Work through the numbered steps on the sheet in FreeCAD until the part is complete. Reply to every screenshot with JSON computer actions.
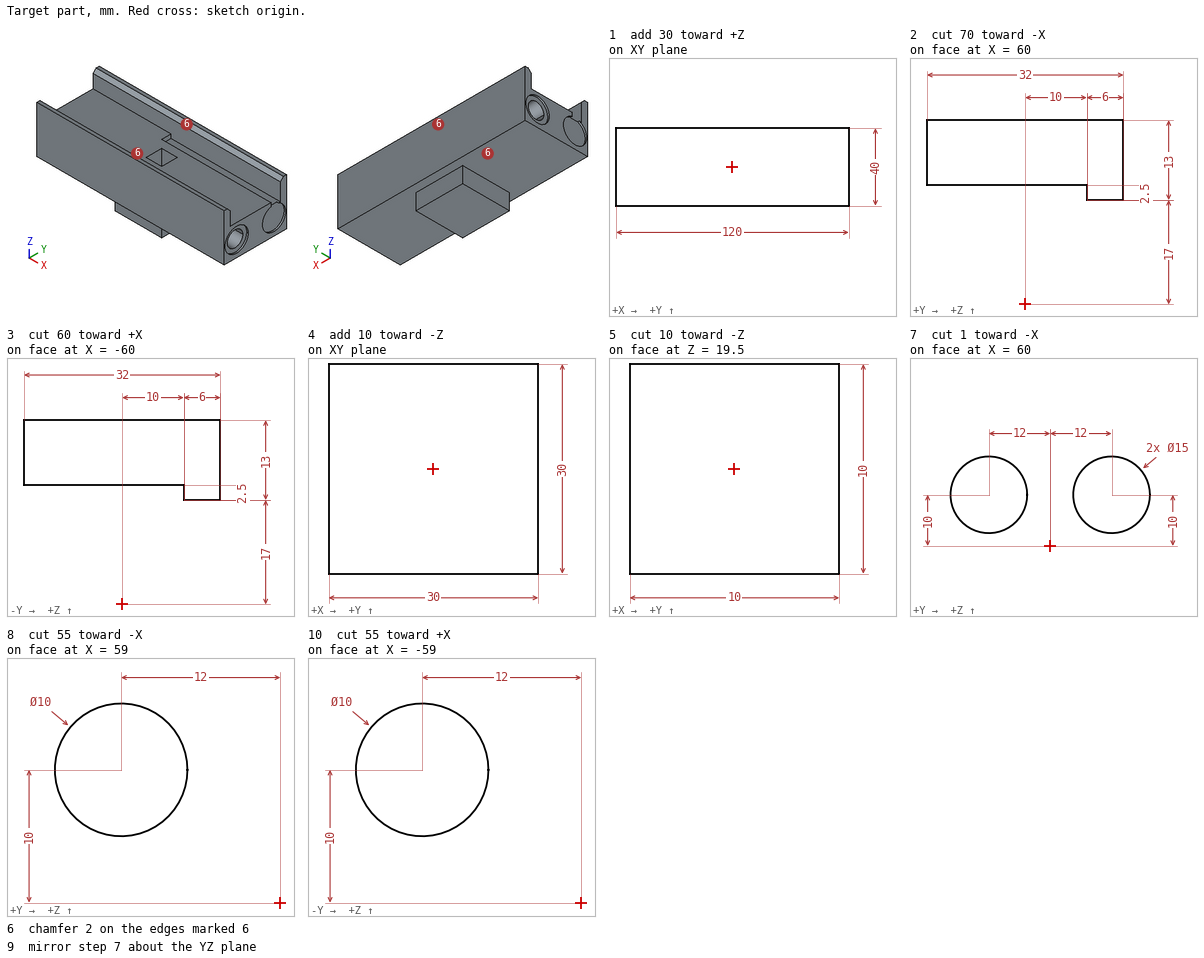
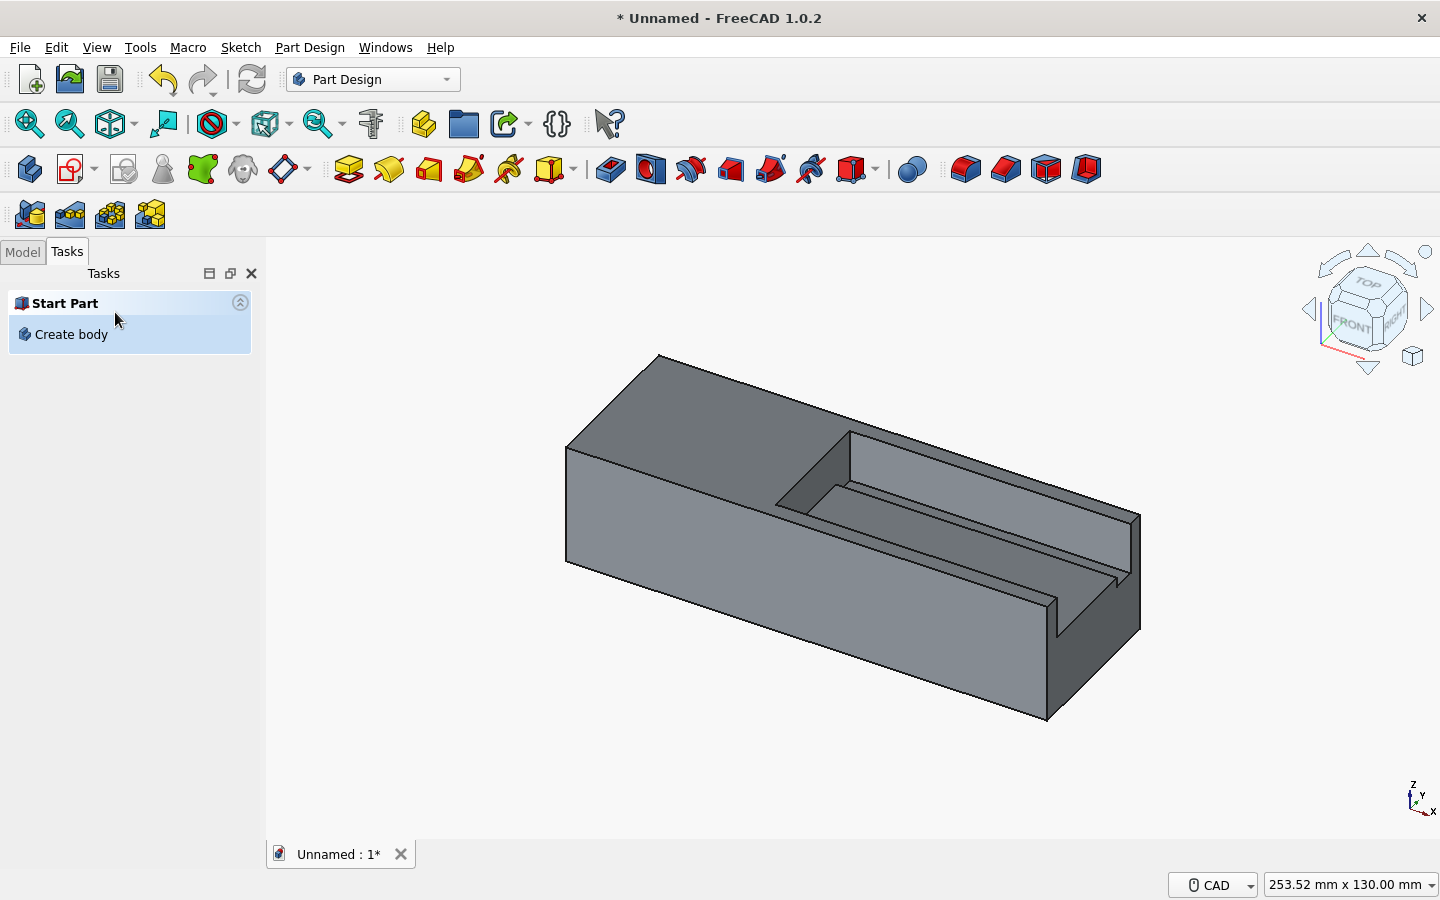
{"action": "key", "text": "6"}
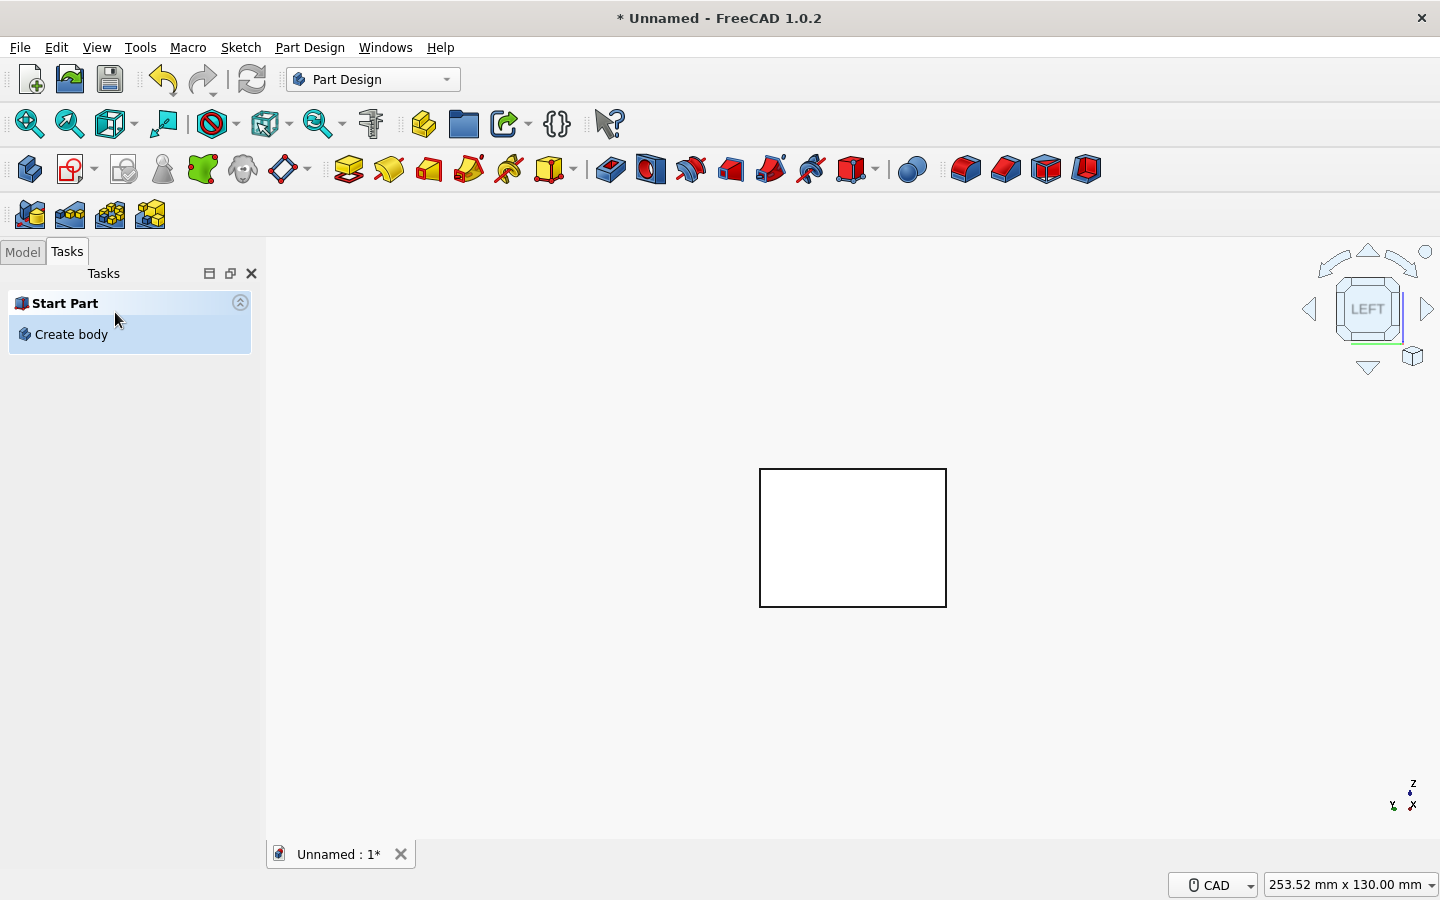
{"action": "left_click", "coordinate": [30, 124]}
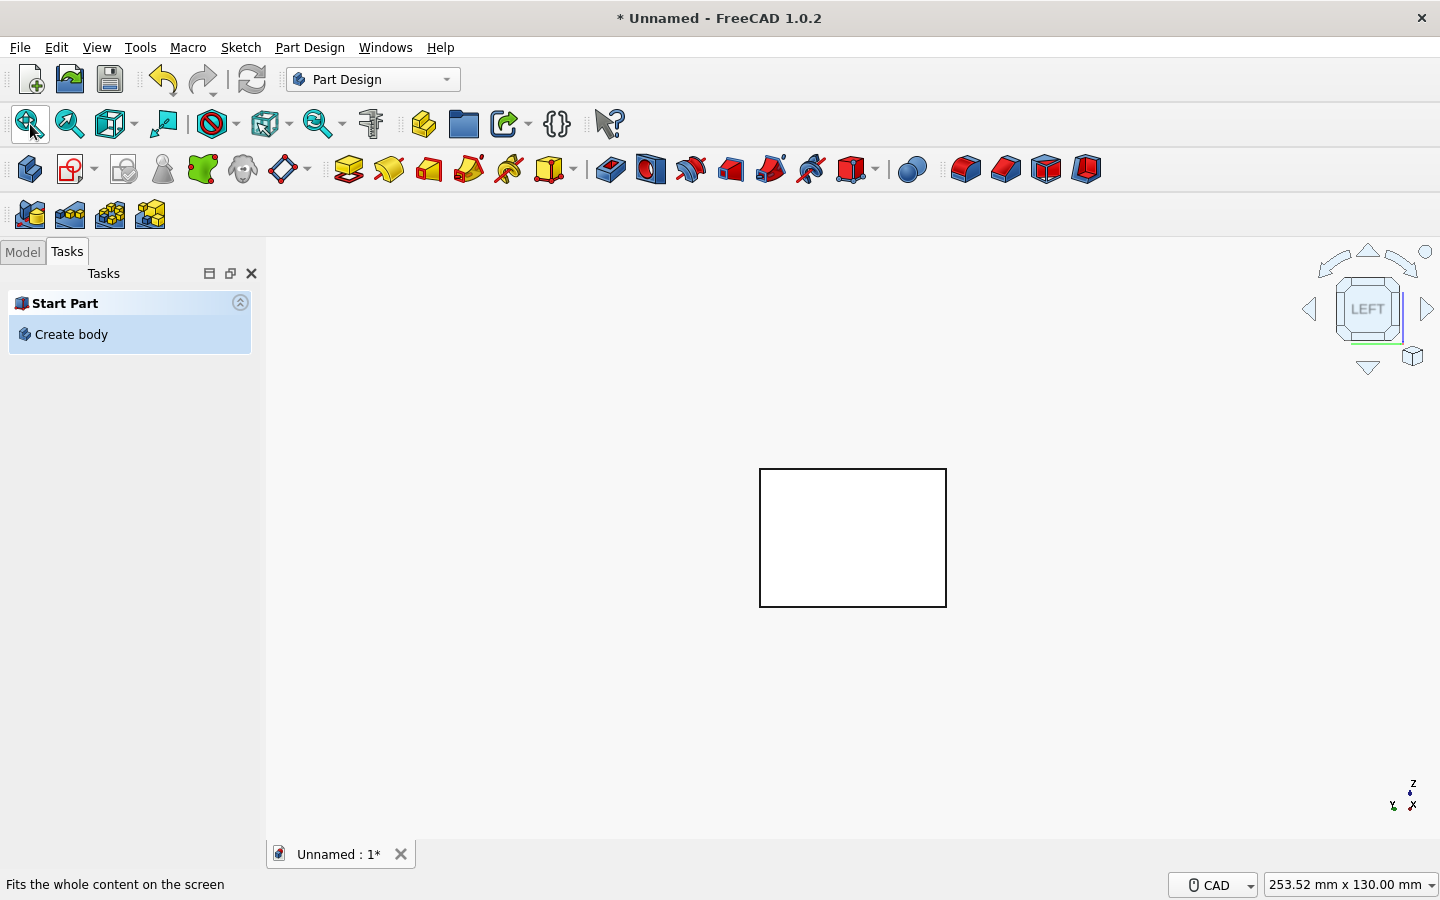
{"action": "left_click", "coordinate": [853, 537]}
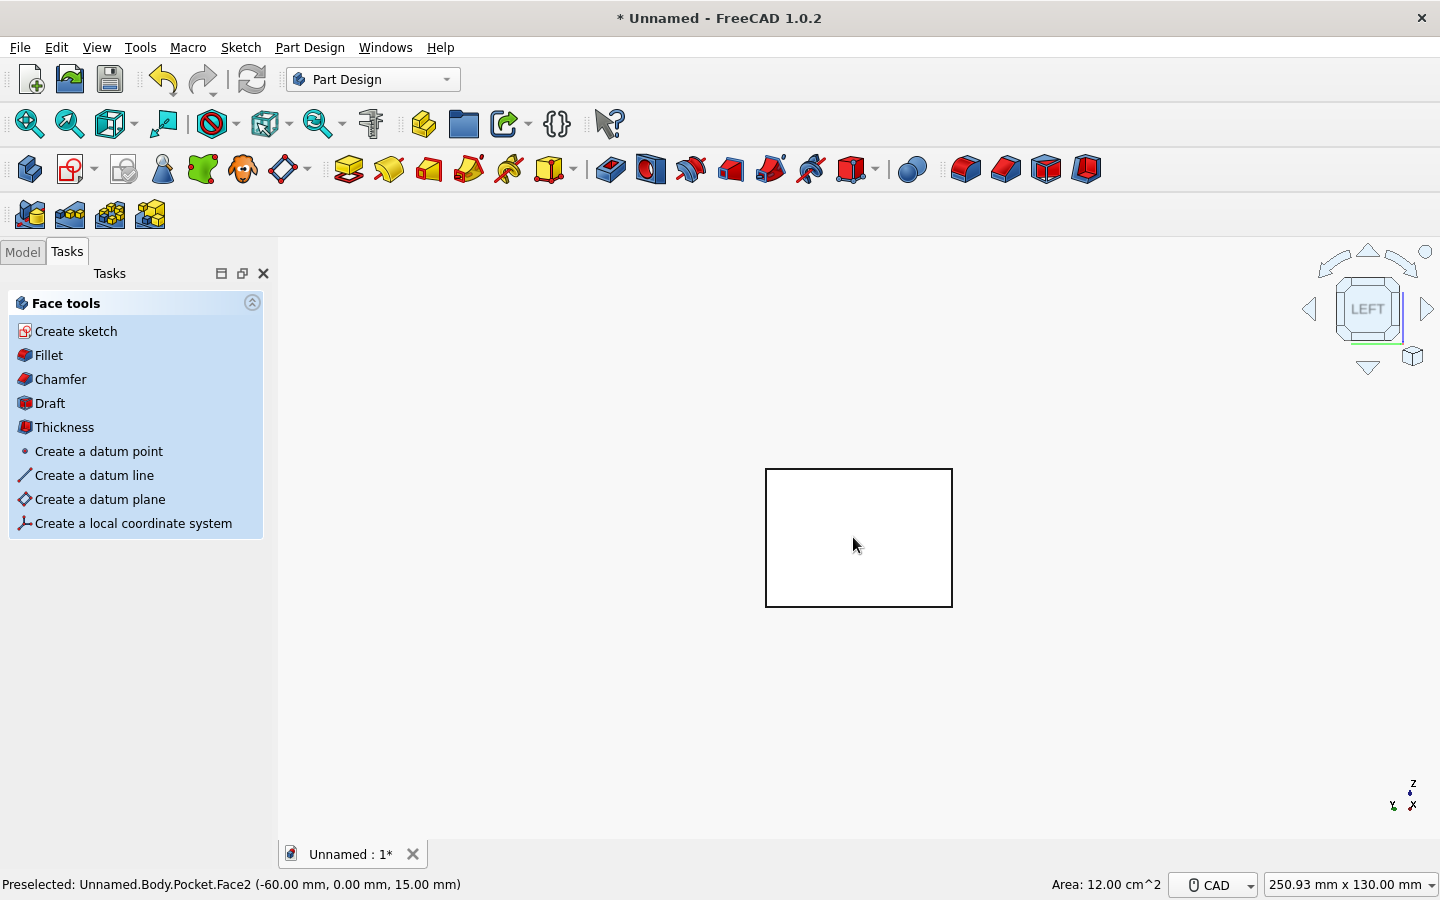
{"action": "left_click", "coordinate": [70, 170]}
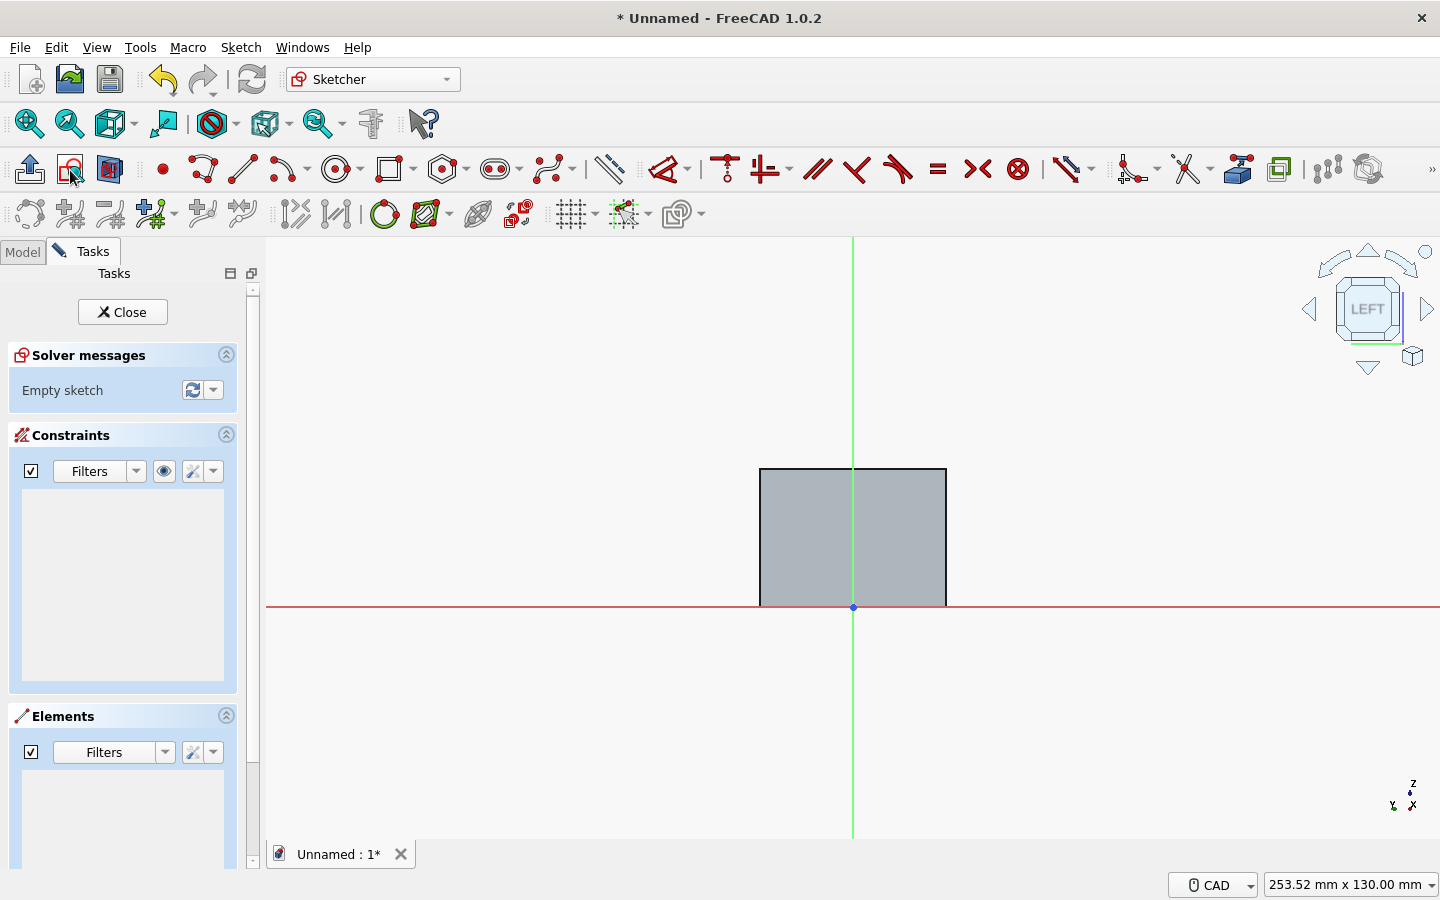
{"action": "scroll", "coordinate": [893, 538], "scroll_direction": "up", "scroll_amount": 5}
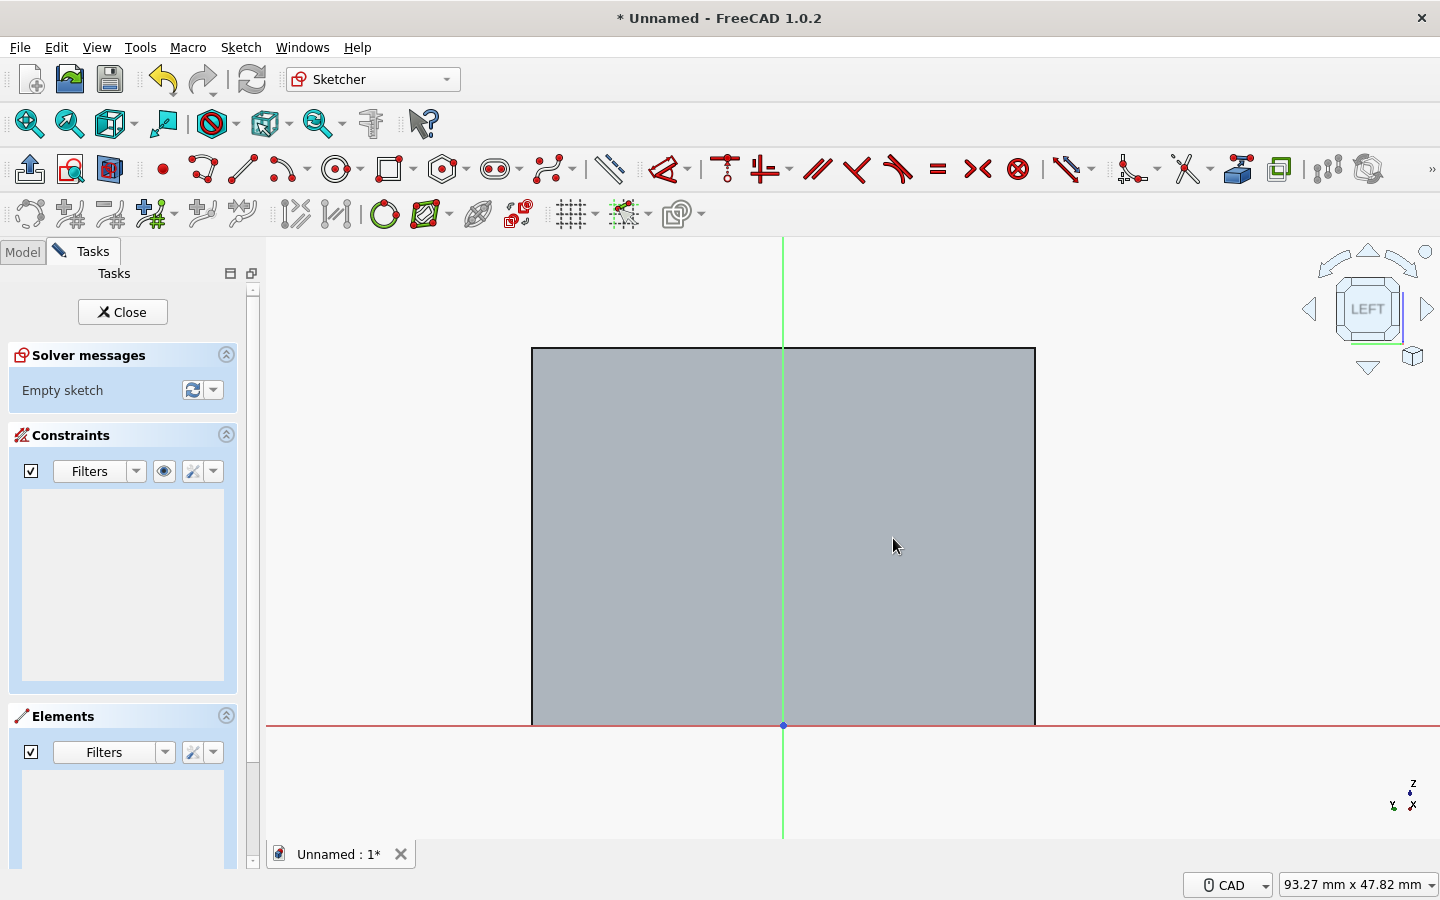
{"action": "key", "text": "g m"}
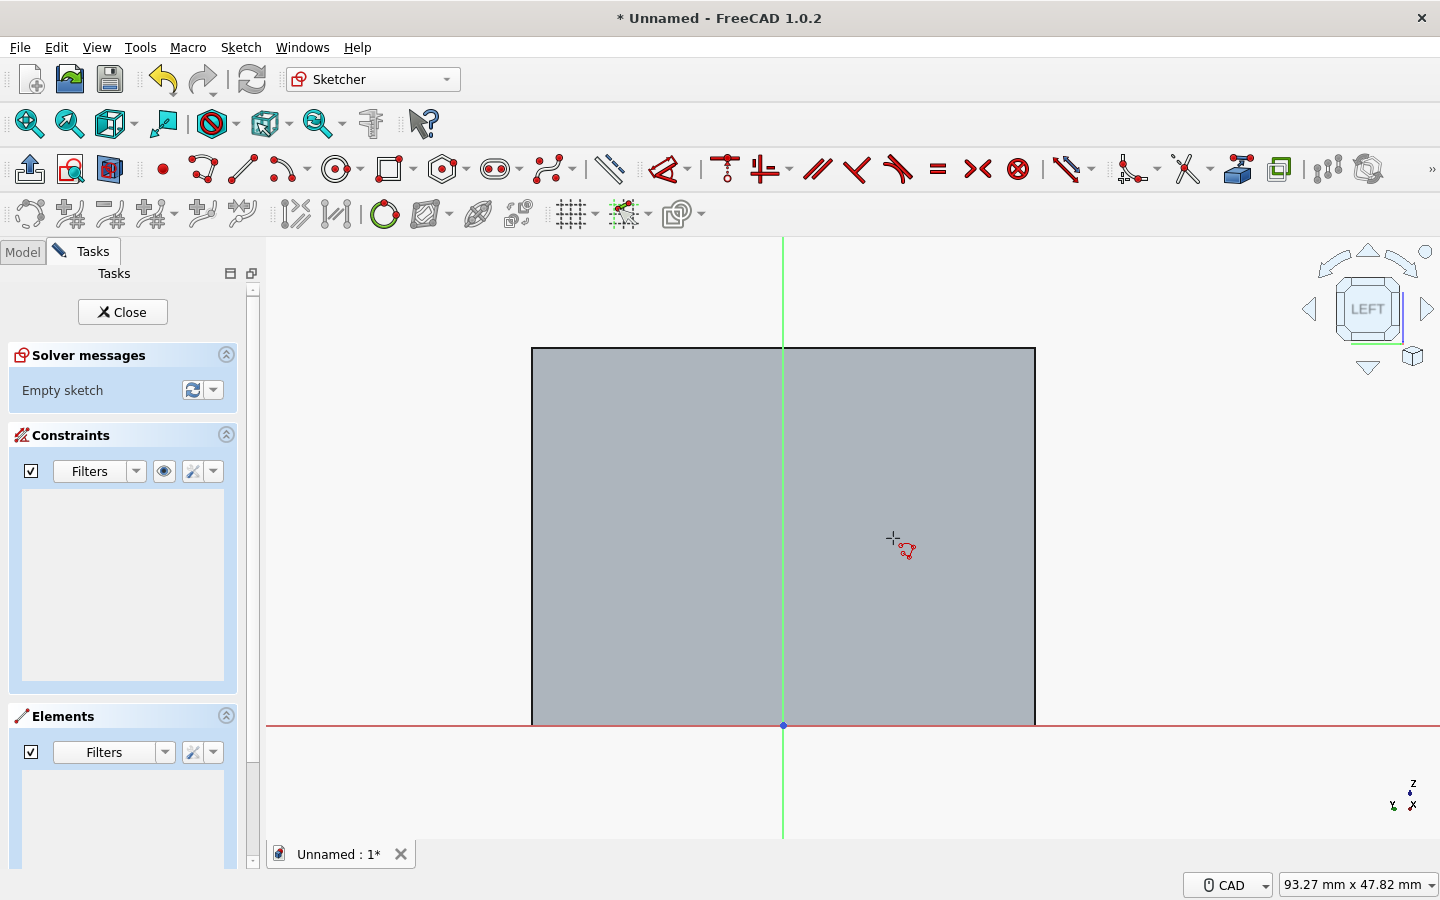
{"action": "left_click", "coordinate": [909, 512]}
{"action": "left_click", "coordinate": [985, 512]}
{"action": "left_click", "coordinate": [985, 348]}
{"action": "left_click", "coordinate": [582, 348]}
{"action": "left_click", "coordinate": [582, 480]}
{"action": "left_click", "coordinate": [909, 480]}
{"action": "left_click", "coordinate": [909, 513]}
{"action": "key", "text": "Escape"}
{"action": "key", "text": "Escape"}